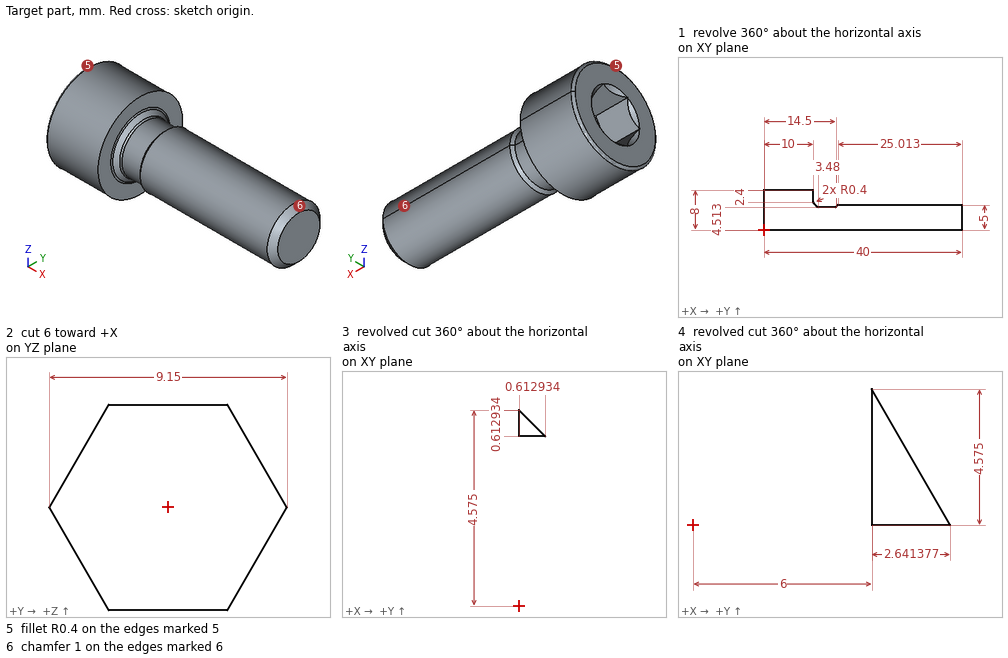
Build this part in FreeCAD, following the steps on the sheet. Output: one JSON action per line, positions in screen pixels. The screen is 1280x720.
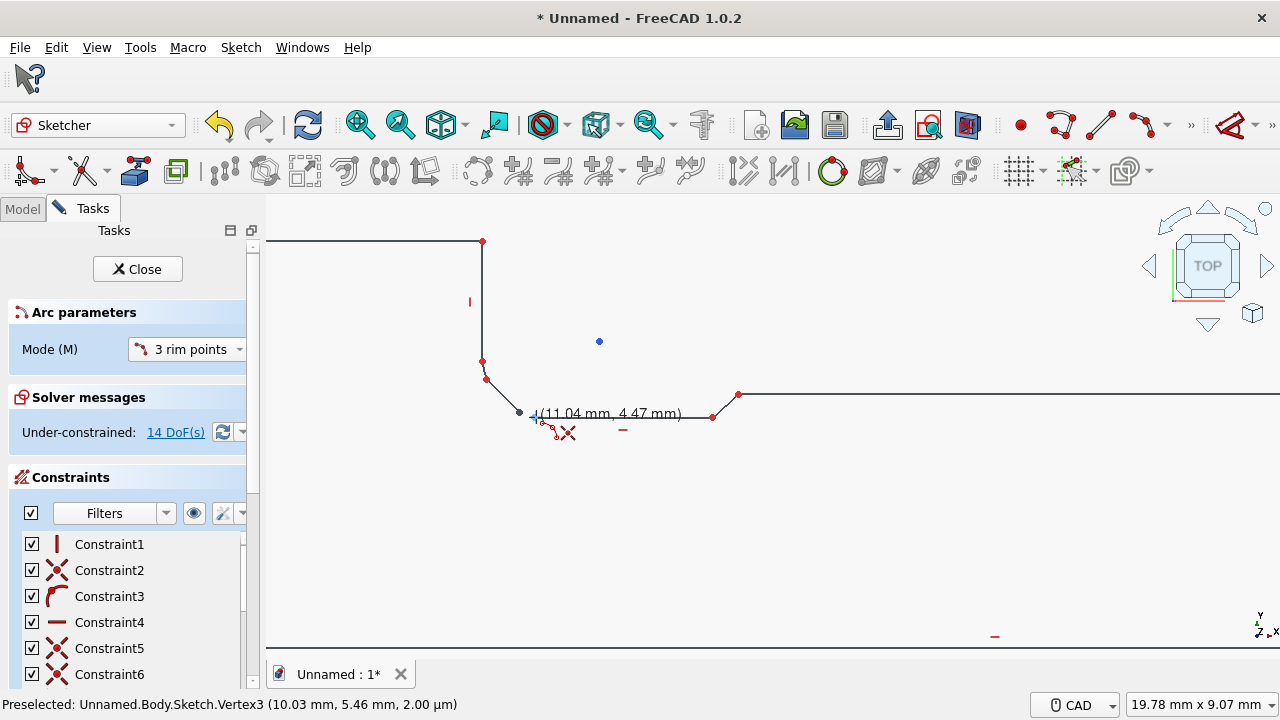
{"action": "left_click", "coordinate": [535, 418]}
{"action": "left_click", "coordinate": [520, 412]}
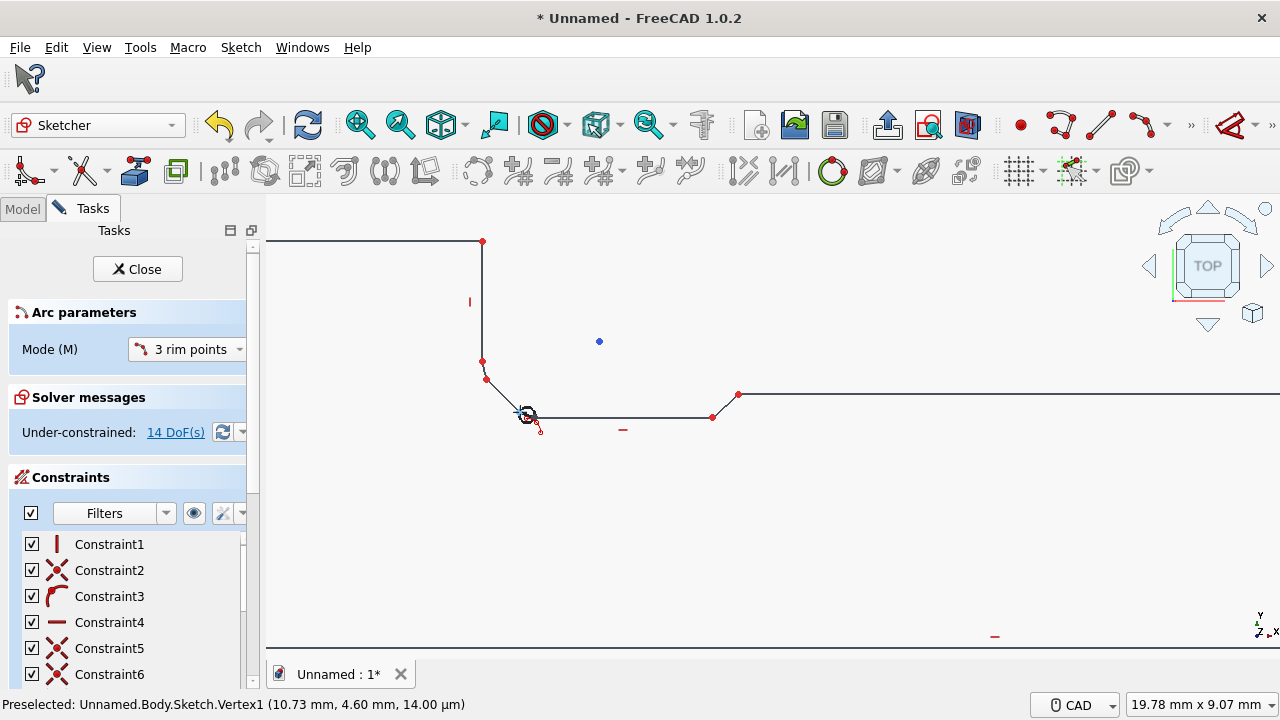
{"action": "scroll", "coordinate": [526, 415], "scroll_direction": "up", "scroll_amount": 11}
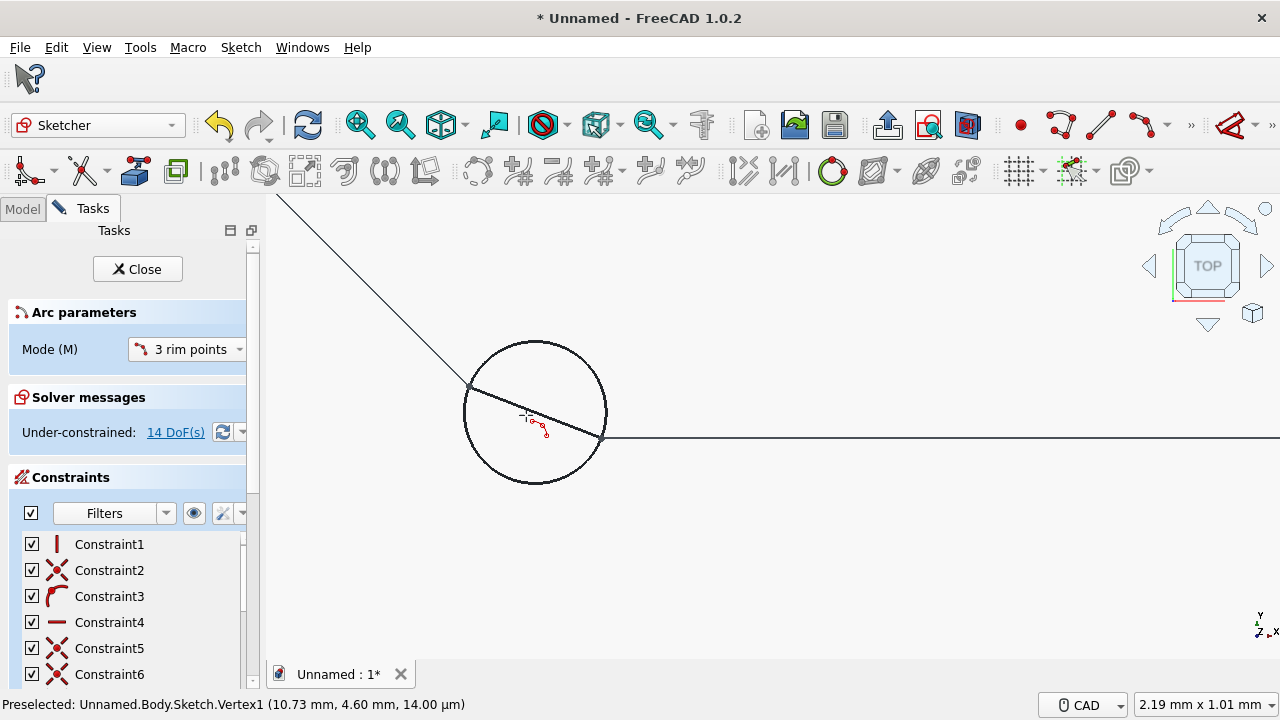
{"action": "left_click", "coordinate": [526, 409]}
{"action": "key", "text": "Escape"}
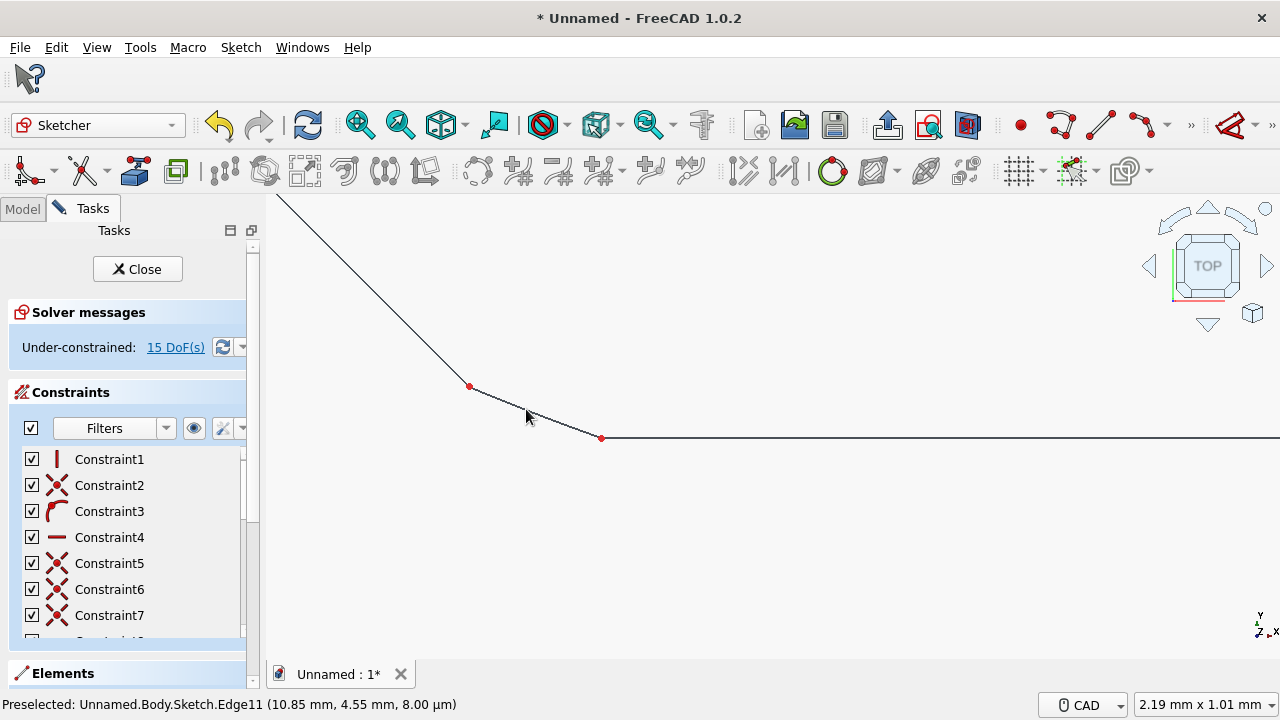
{"action": "scroll", "coordinate": [532, 416], "scroll_direction": "down", "scroll_amount": 16}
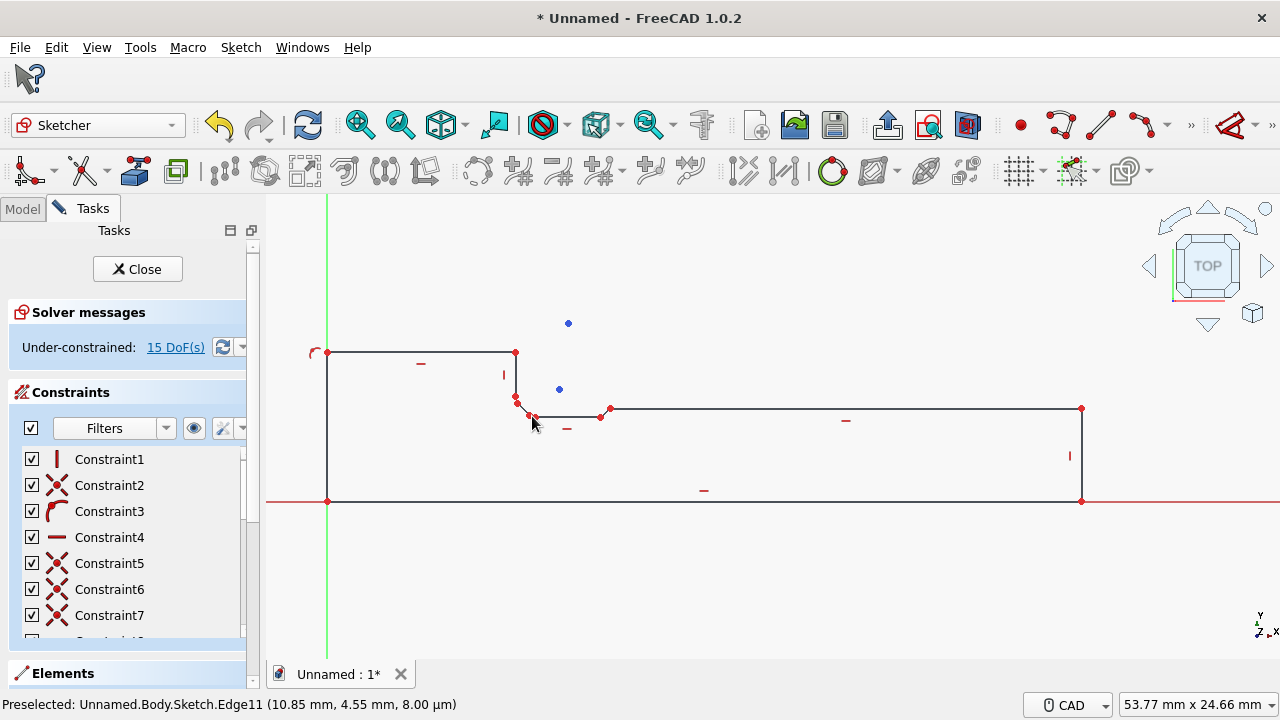
{"action": "scroll", "coordinate": [526, 412], "scroll_direction": "up", "scroll_amount": 5}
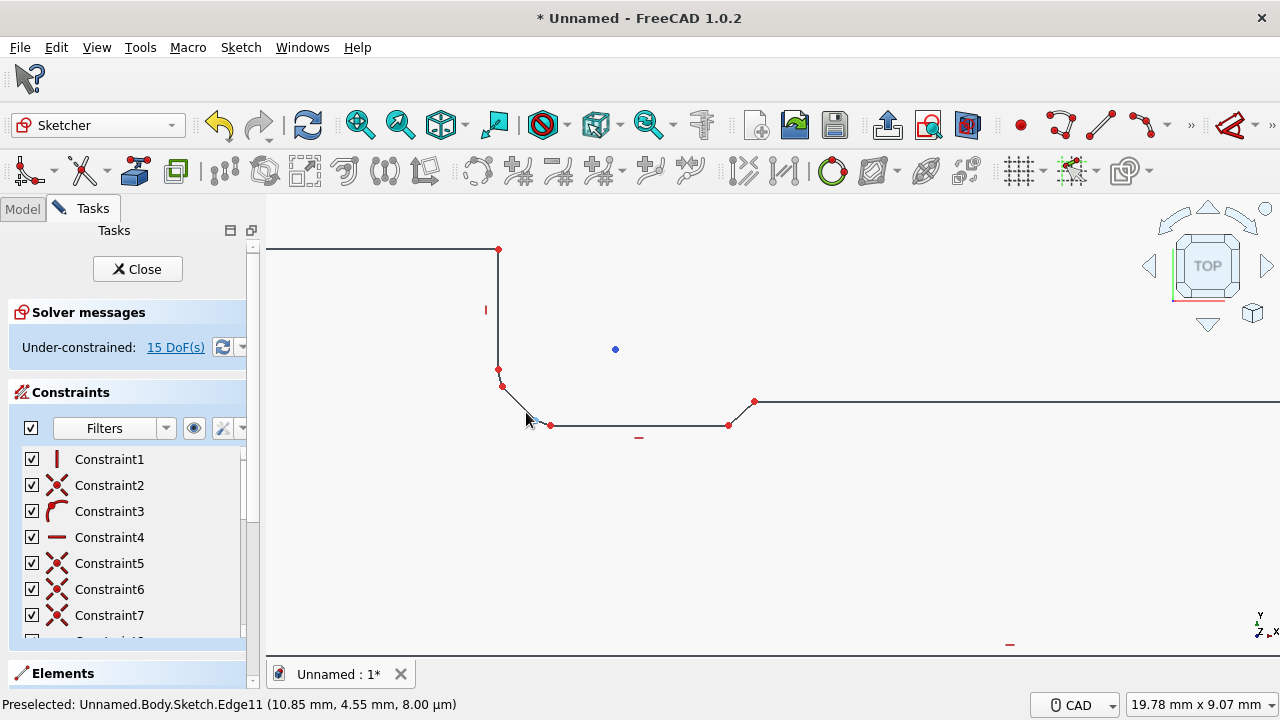
{"action": "left_click", "coordinate": [526, 410]}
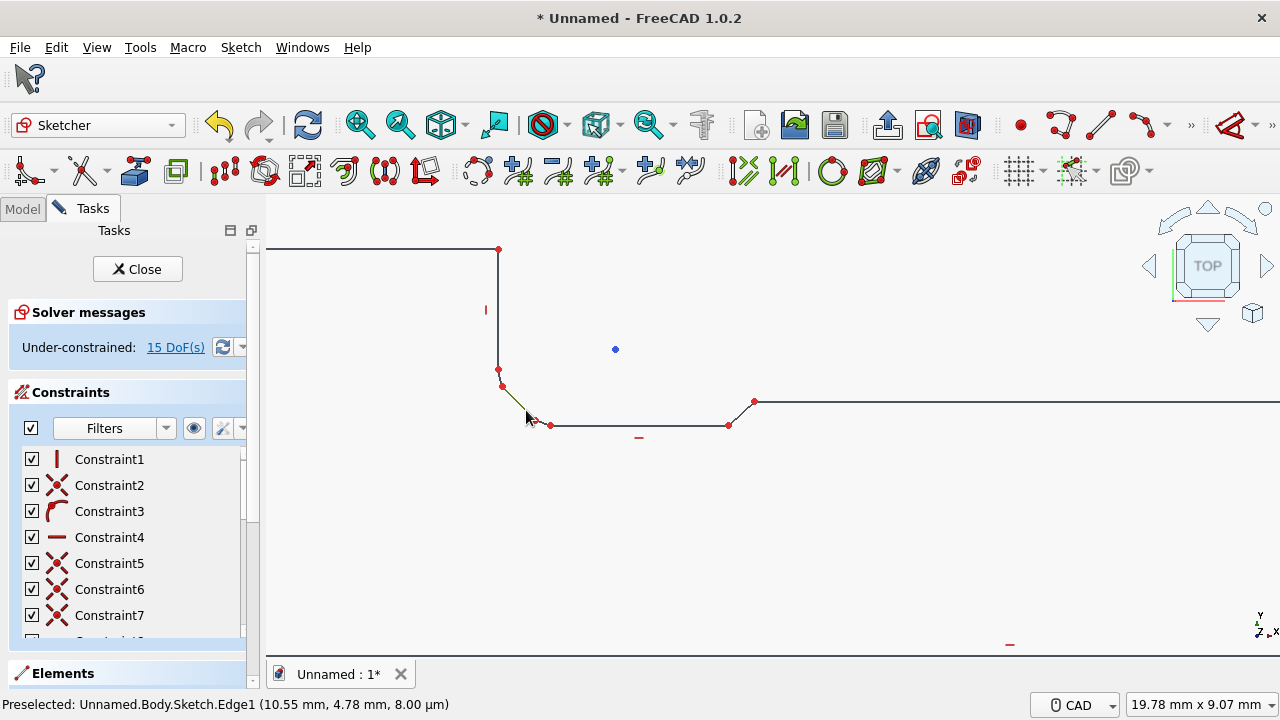
{"action": "scroll", "coordinate": [500, 378], "scroll_direction": "up", "scroll_amount": 3}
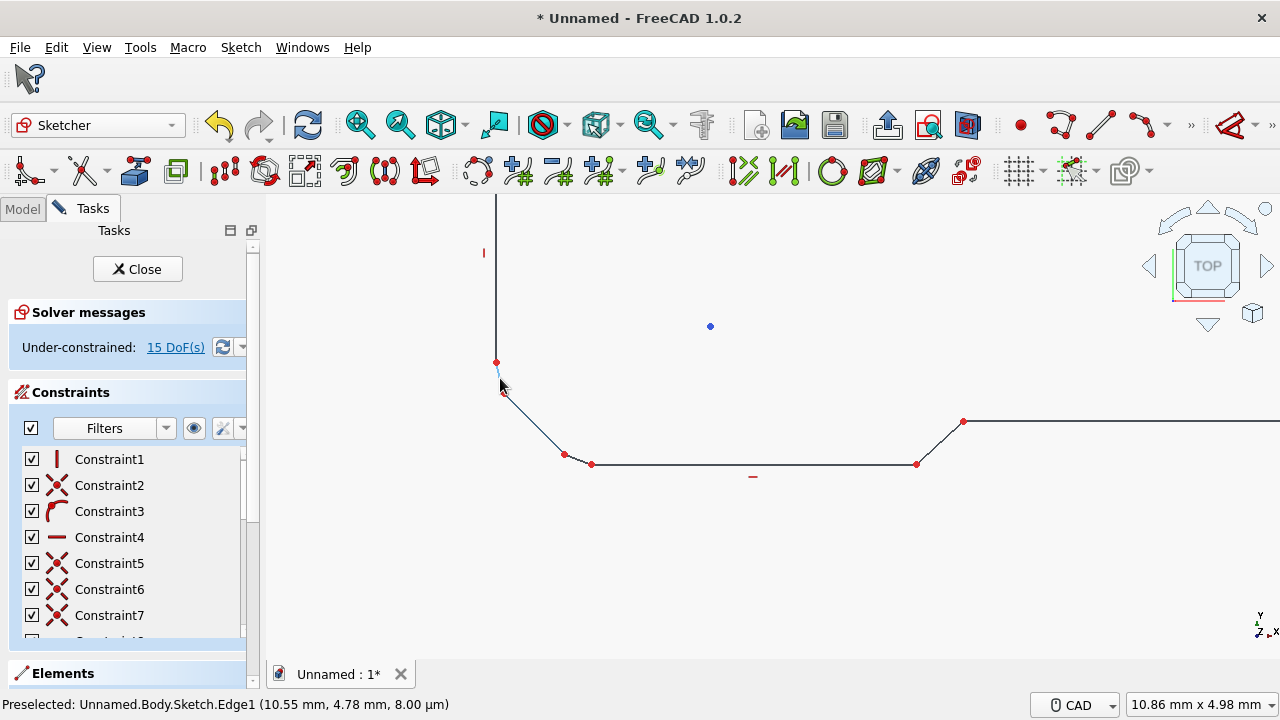
{"action": "left_click", "coordinate": [500, 378]}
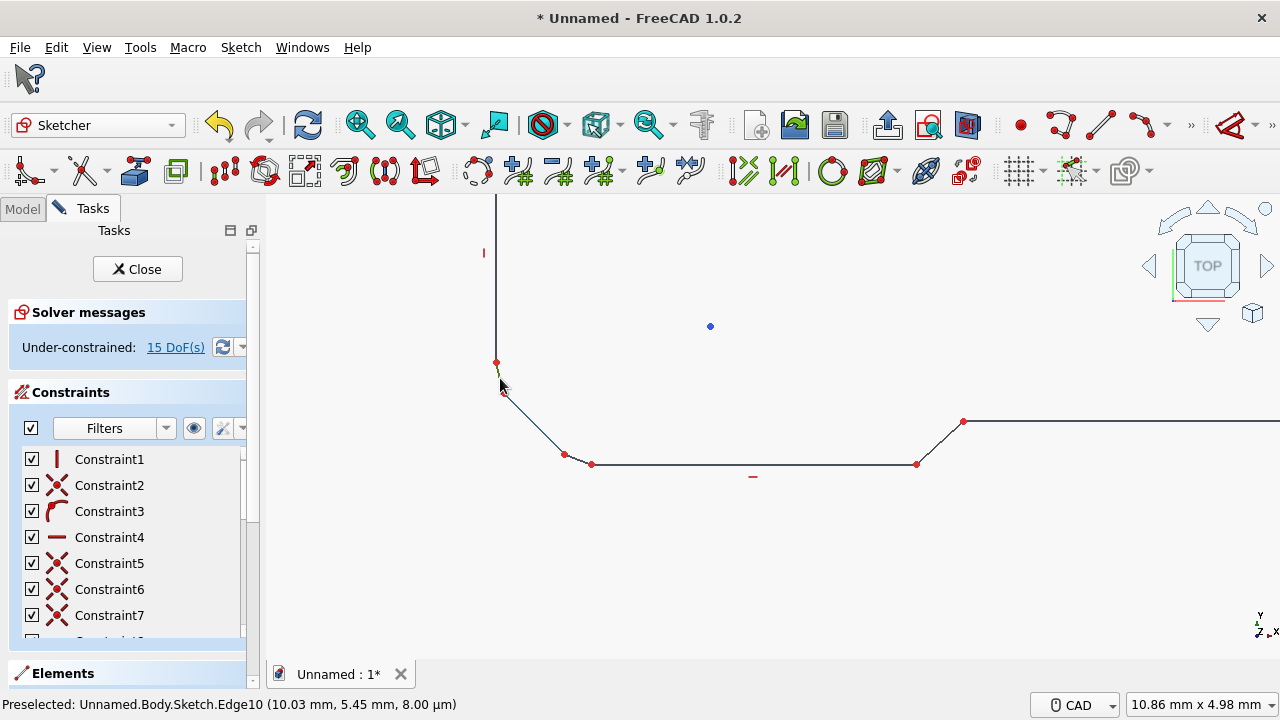
{"action": "key", "text": "t"}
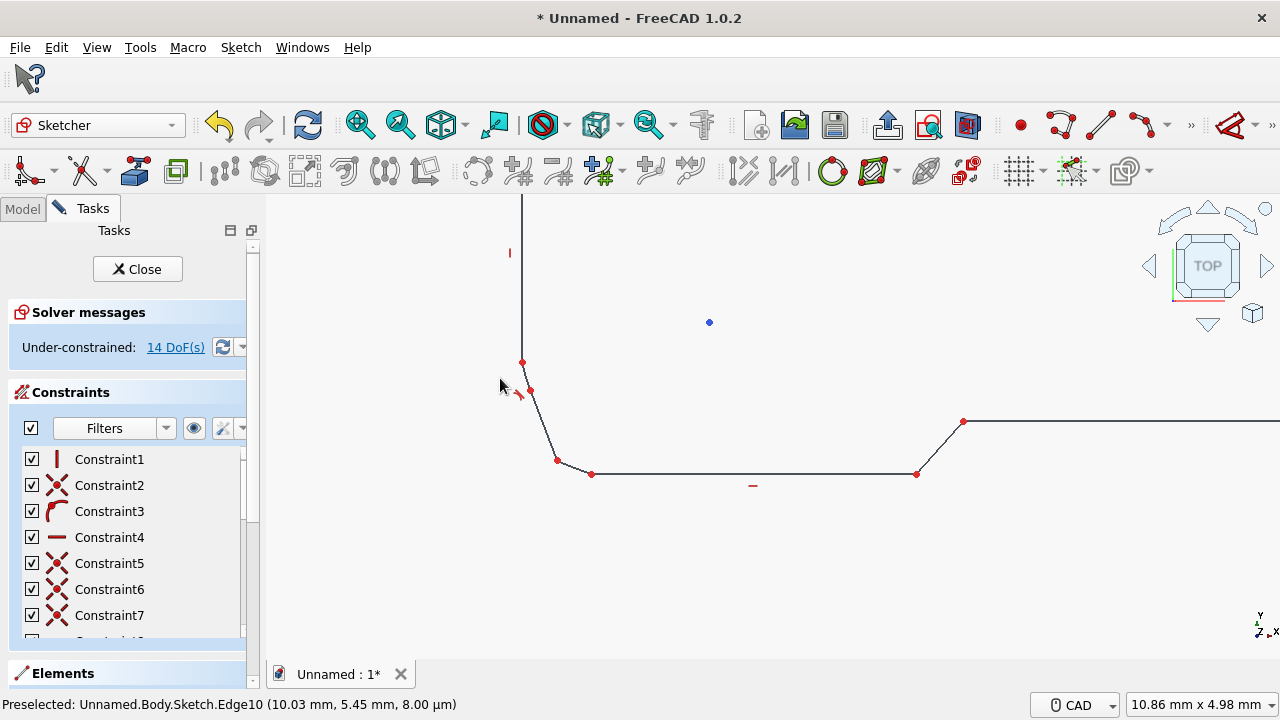
{"action": "left_click", "coordinate": [549, 440]}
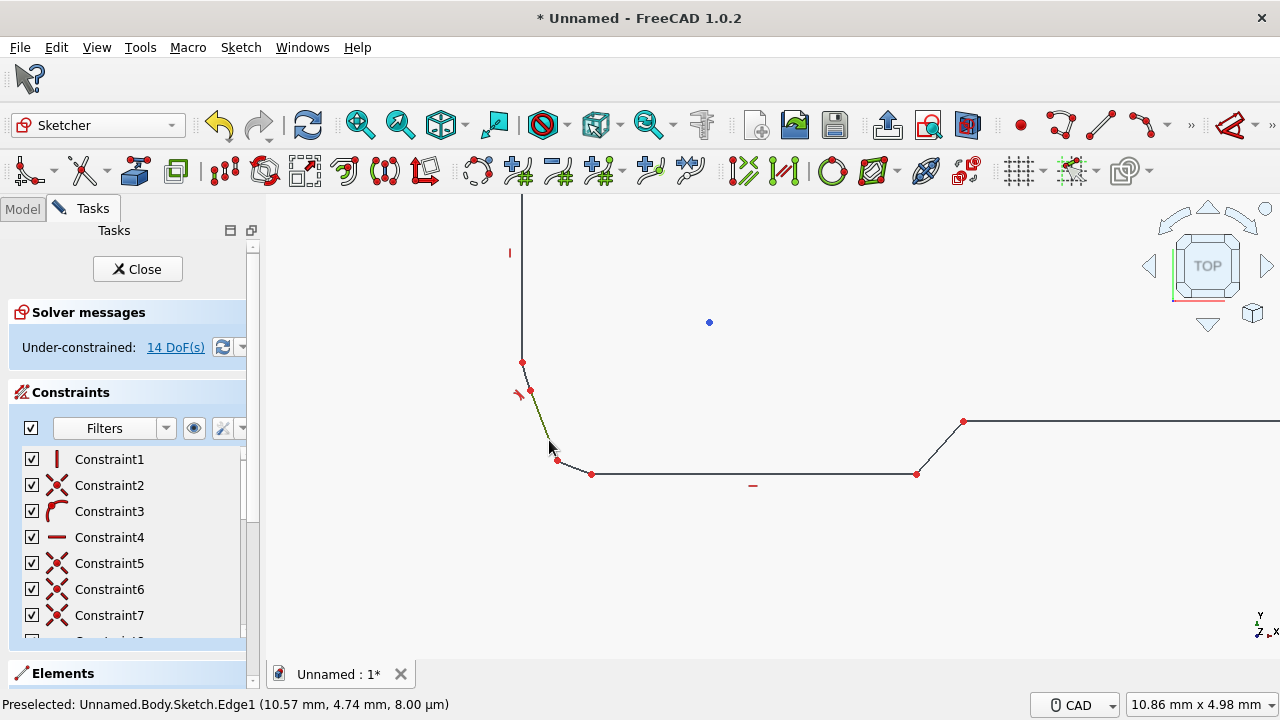
{"action": "scroll", "coordinate": [567, 465], "scroll_direction": "up", "scroll_amount": 2}